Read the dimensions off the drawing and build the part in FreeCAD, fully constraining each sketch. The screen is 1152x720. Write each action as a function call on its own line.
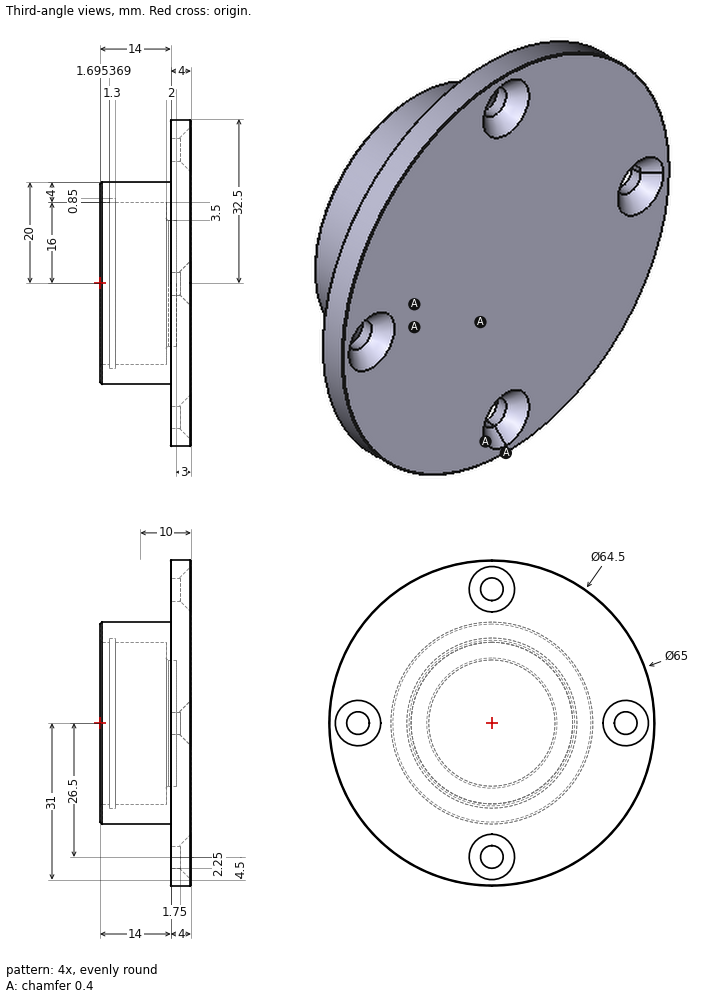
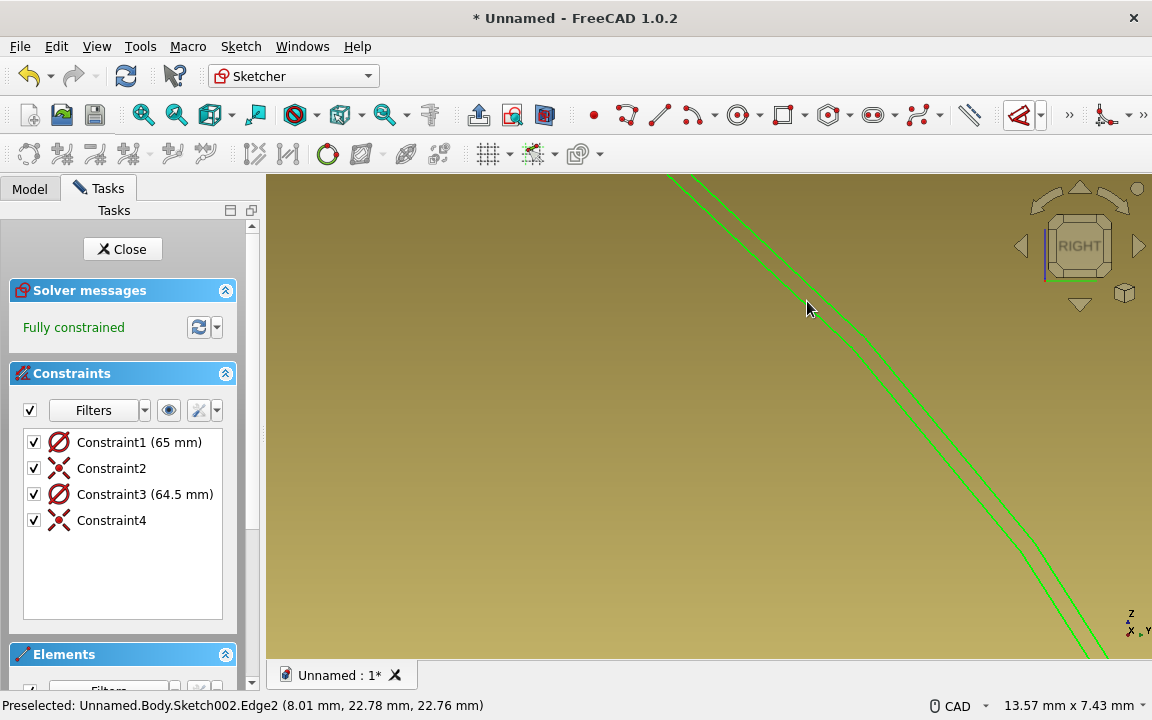
click(123, 249)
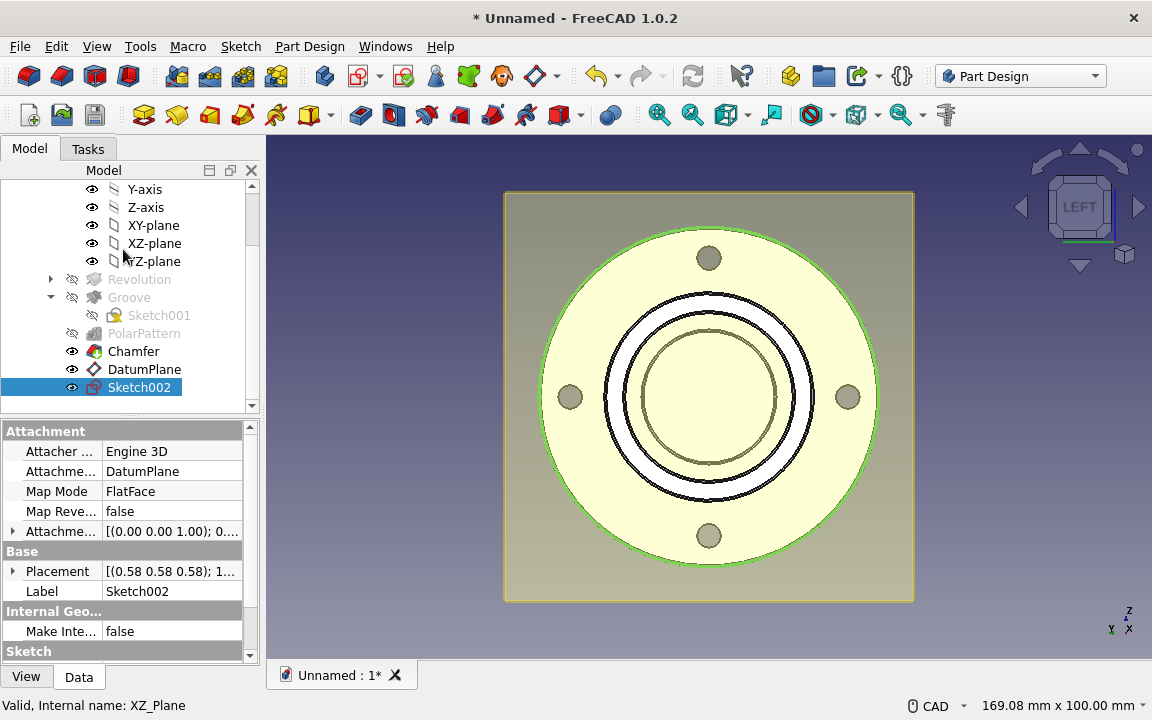
click(361, 116)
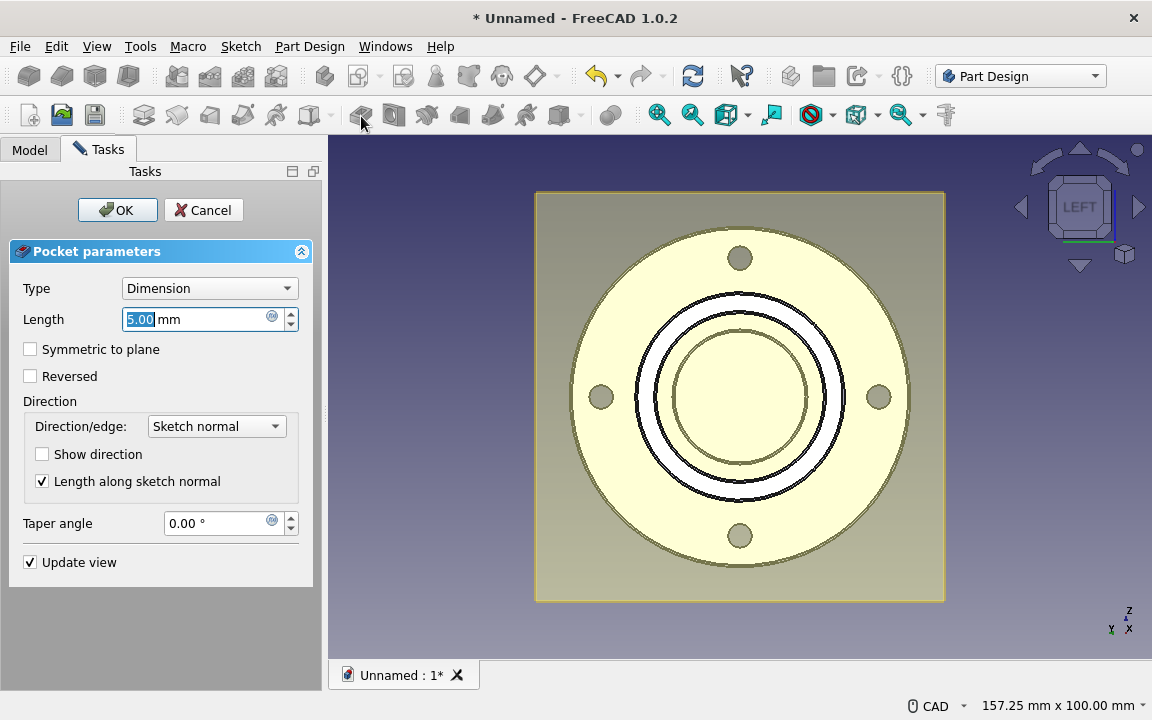
text(10)
key(Tab)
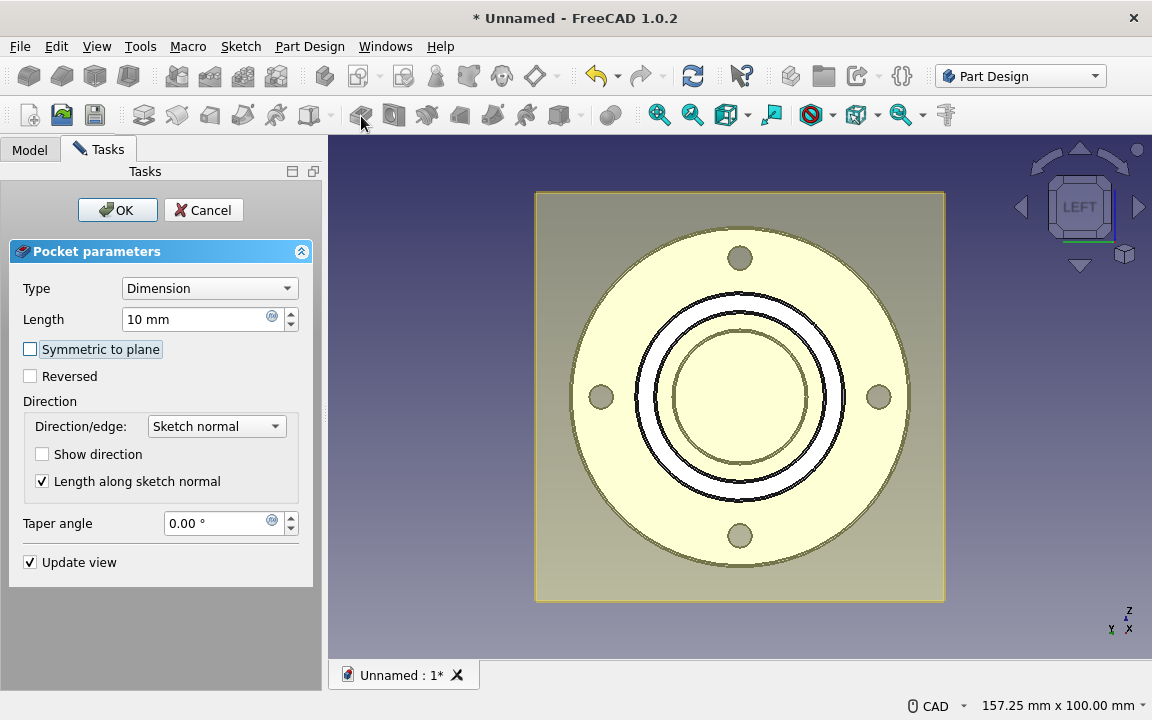
click(31, 376)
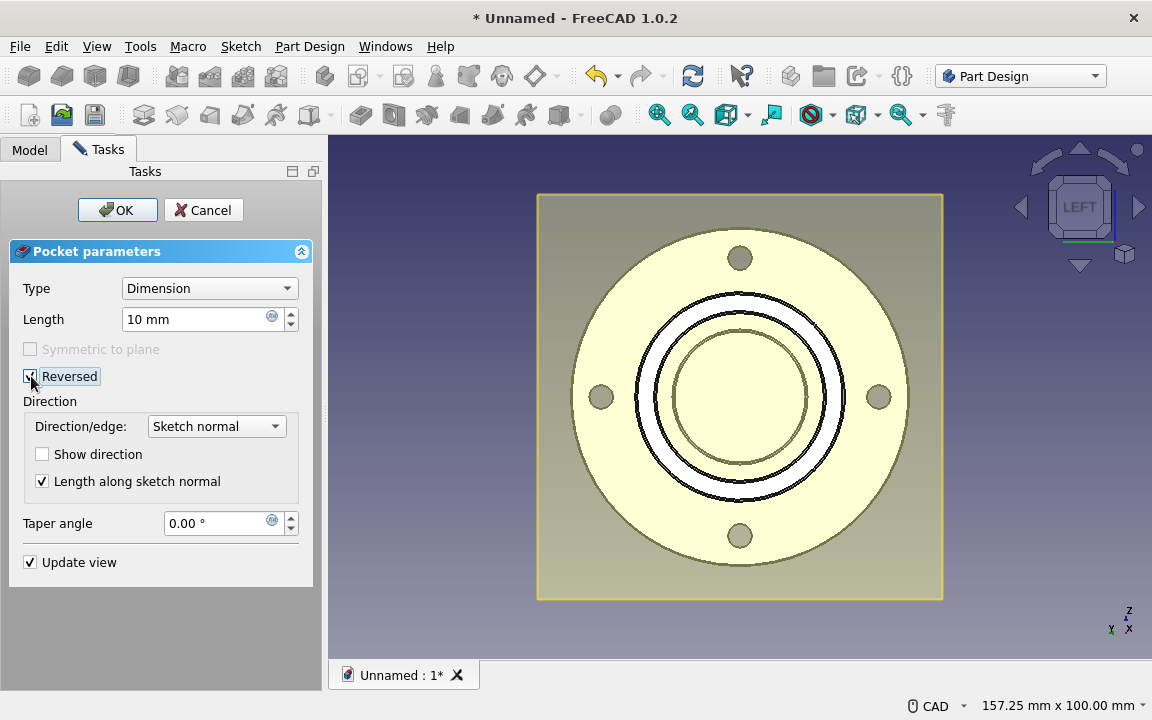
click(118, 210)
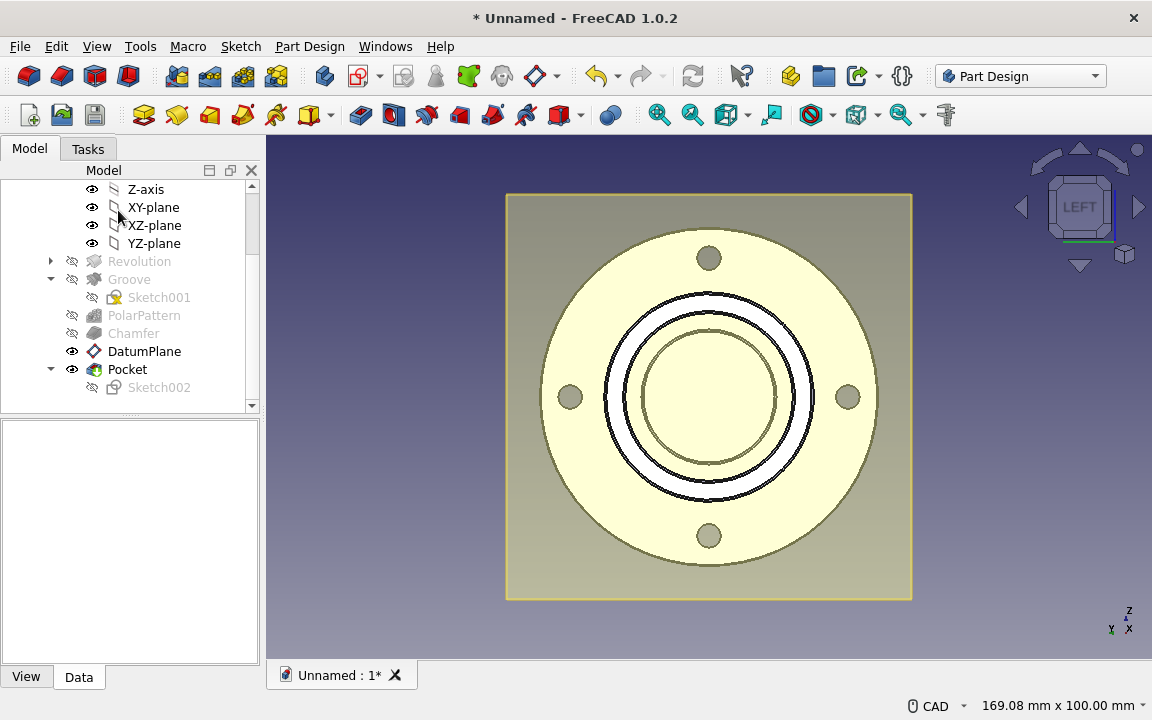
click(117, 351)
key(space)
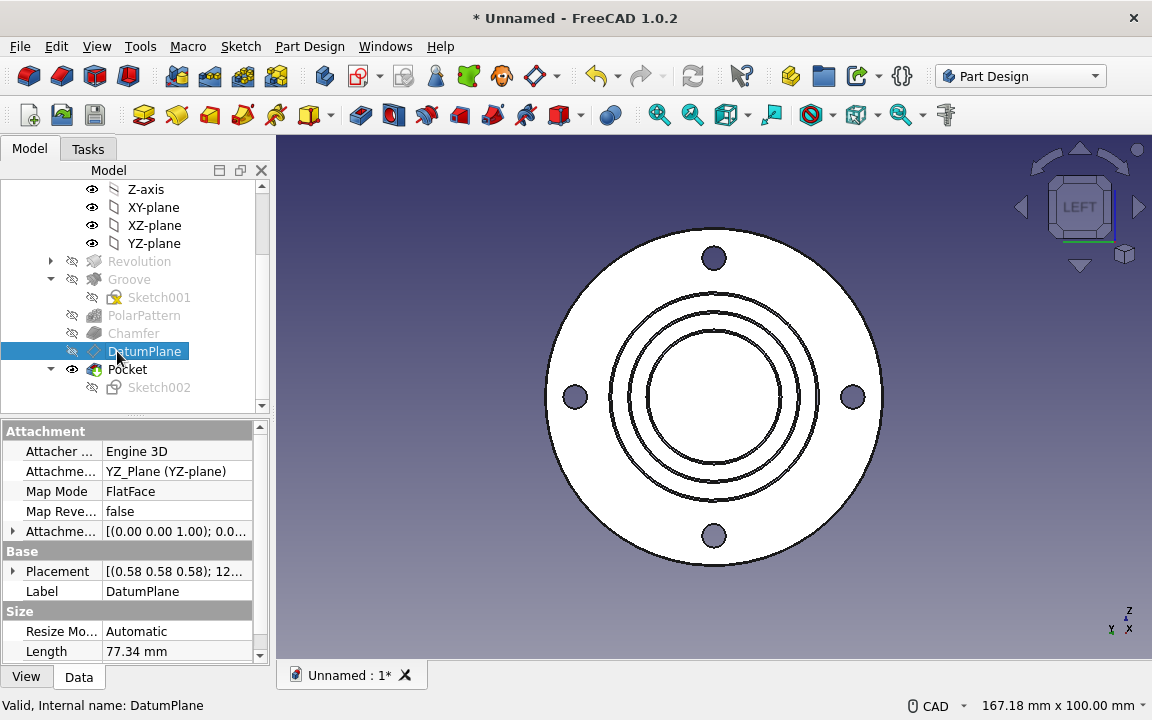
key(0)